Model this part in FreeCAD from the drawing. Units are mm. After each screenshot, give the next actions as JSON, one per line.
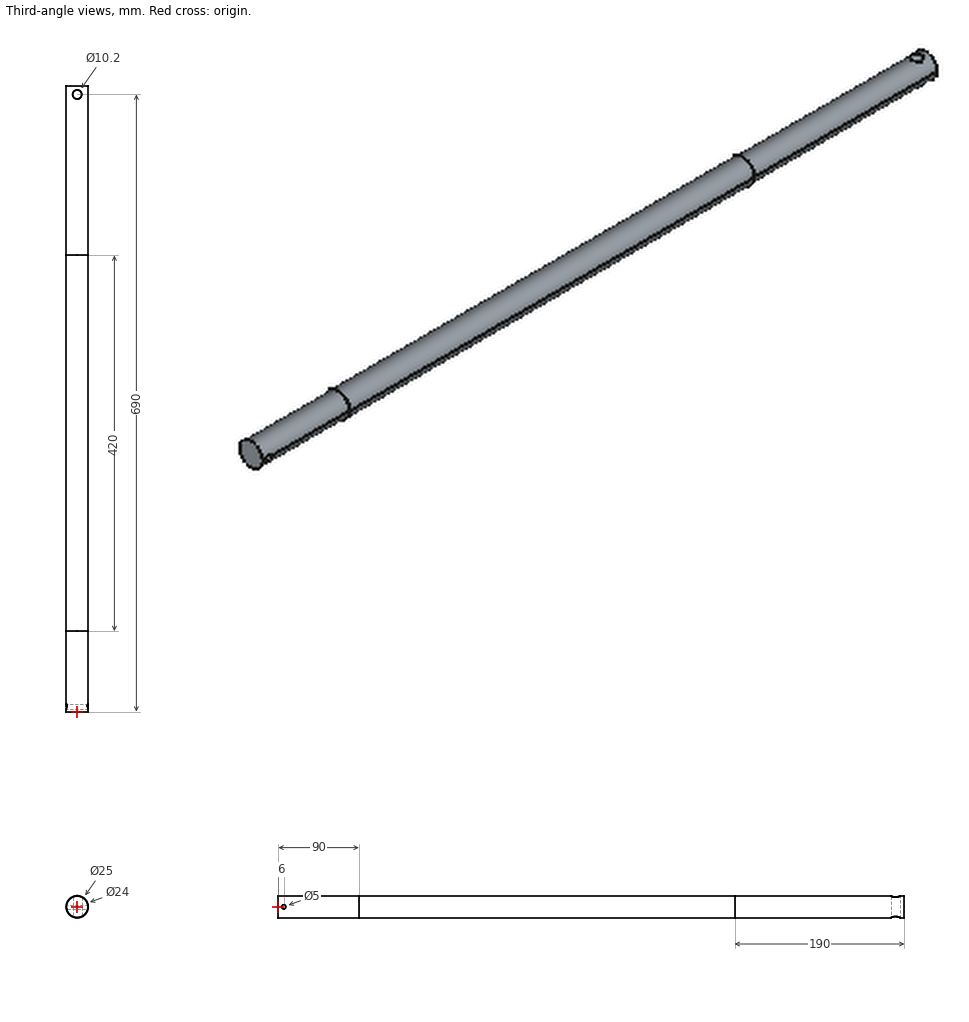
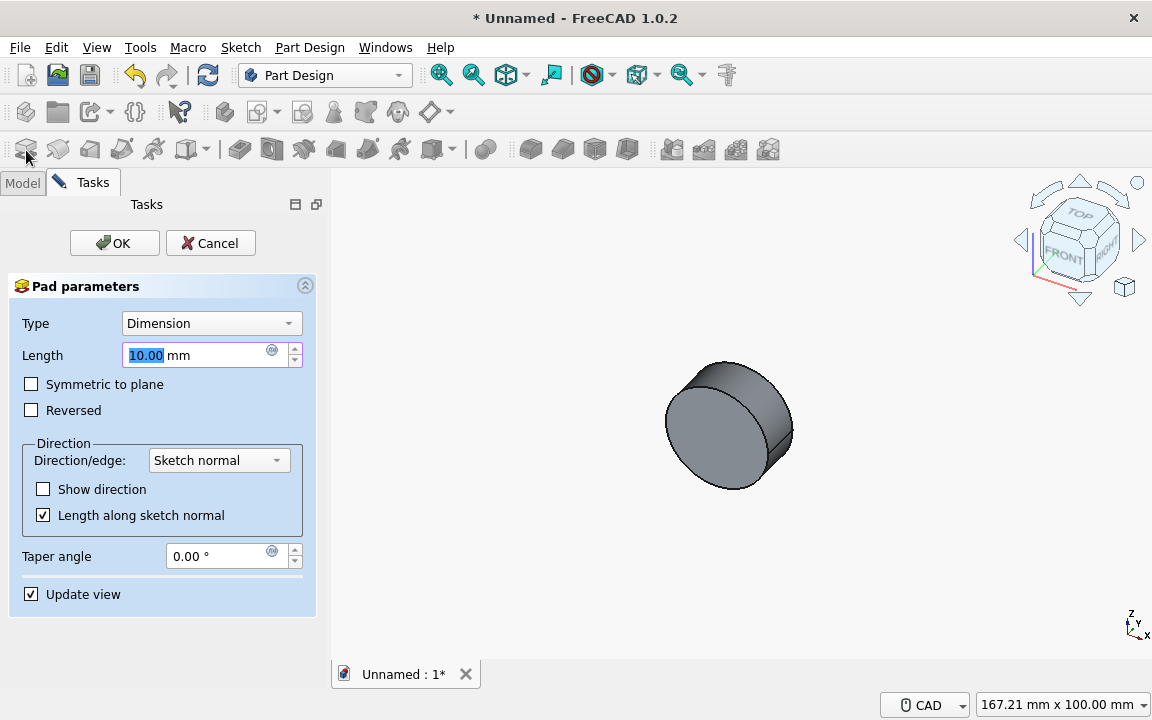
{"action": "type", "text": "90"}
{"action": "key", "text": "Tab"}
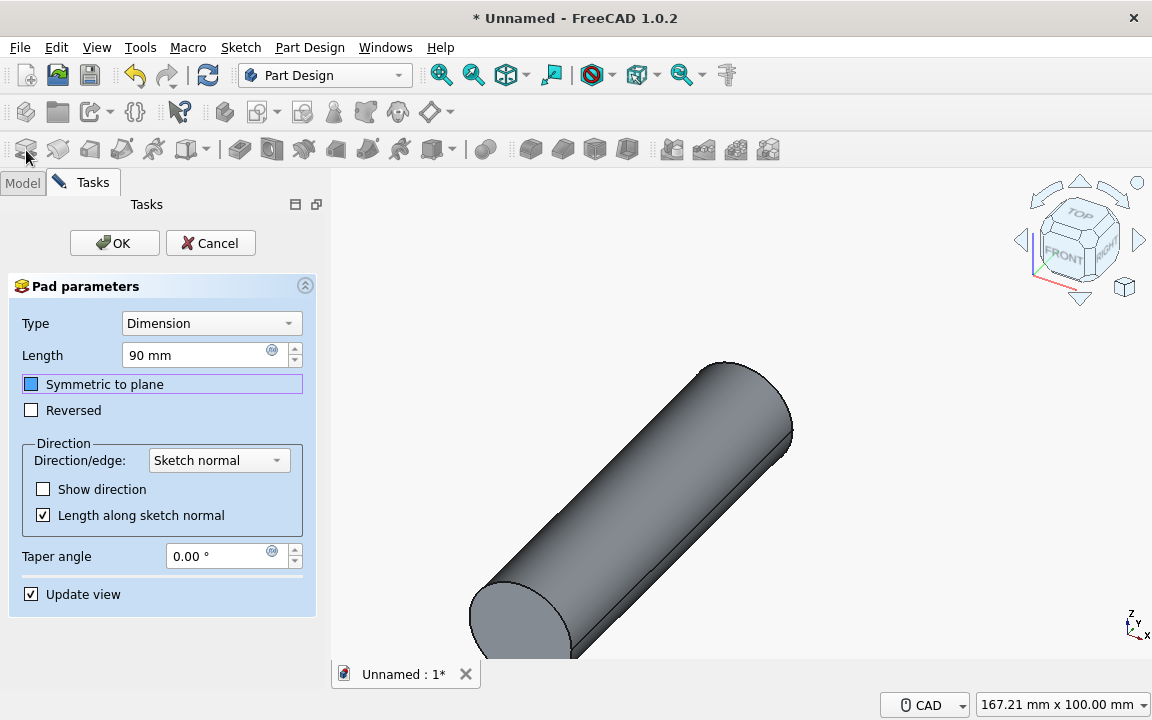
{"action": "left_click", "coordinate": [30, 410]}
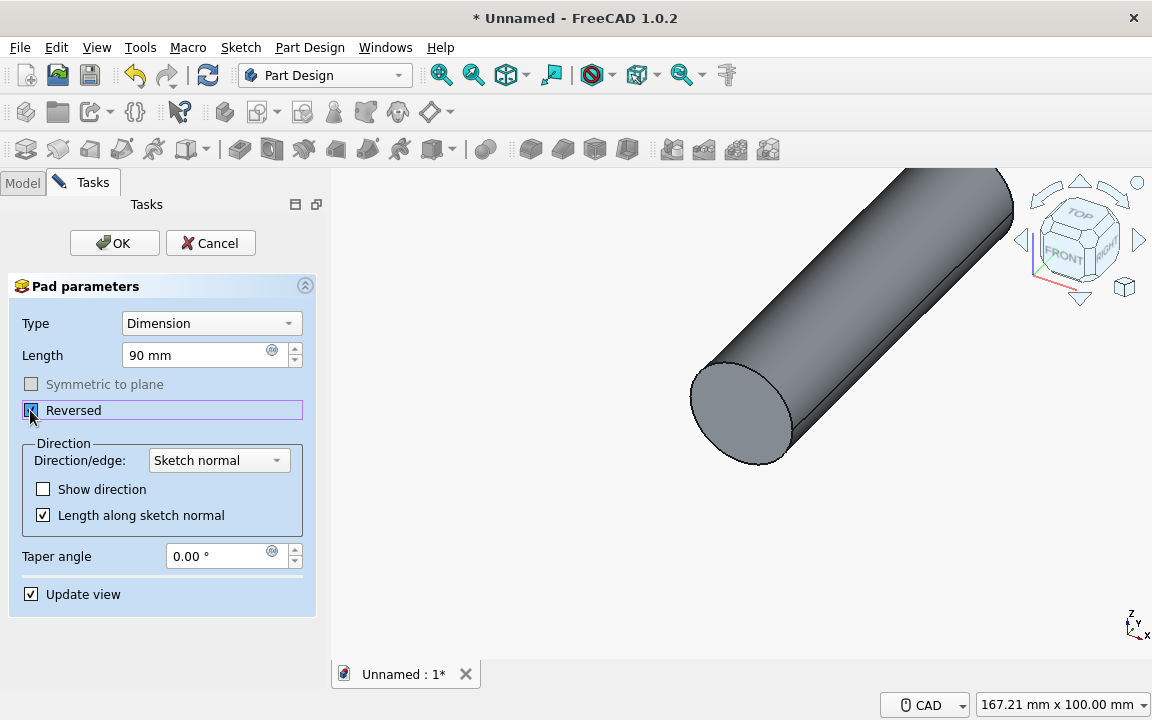
{"action": "left_click", "coordinate": [115, 243]}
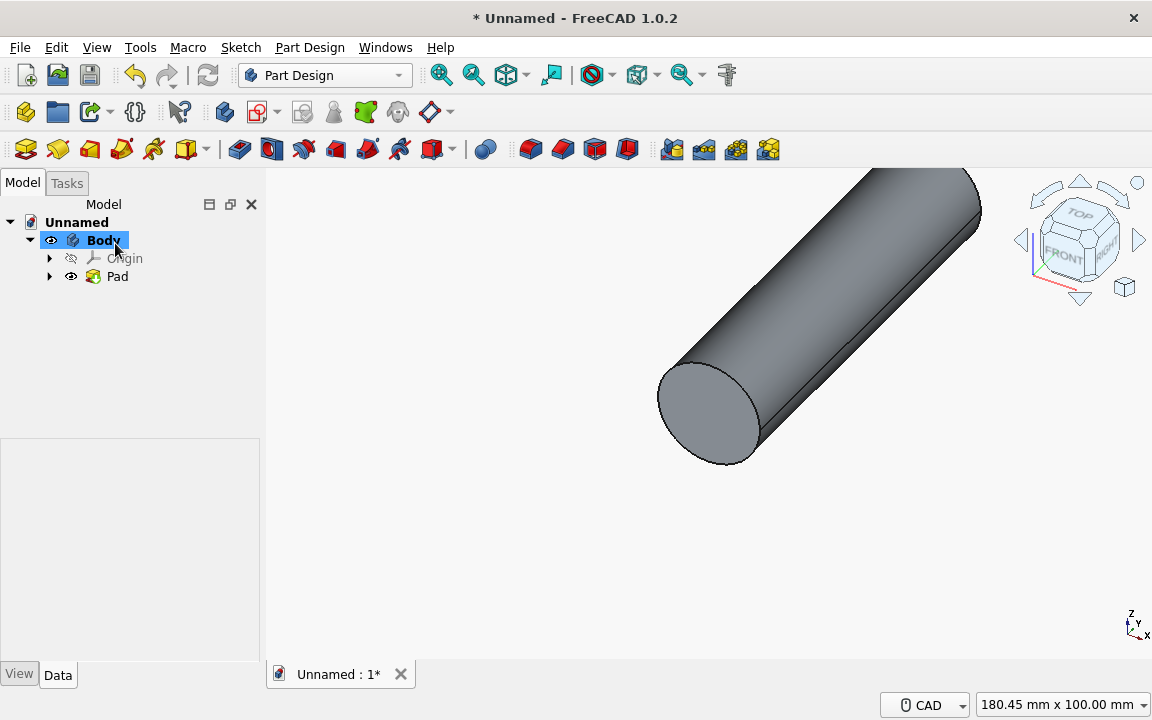
{"action": "left_click", "coordinate": [442, 76]}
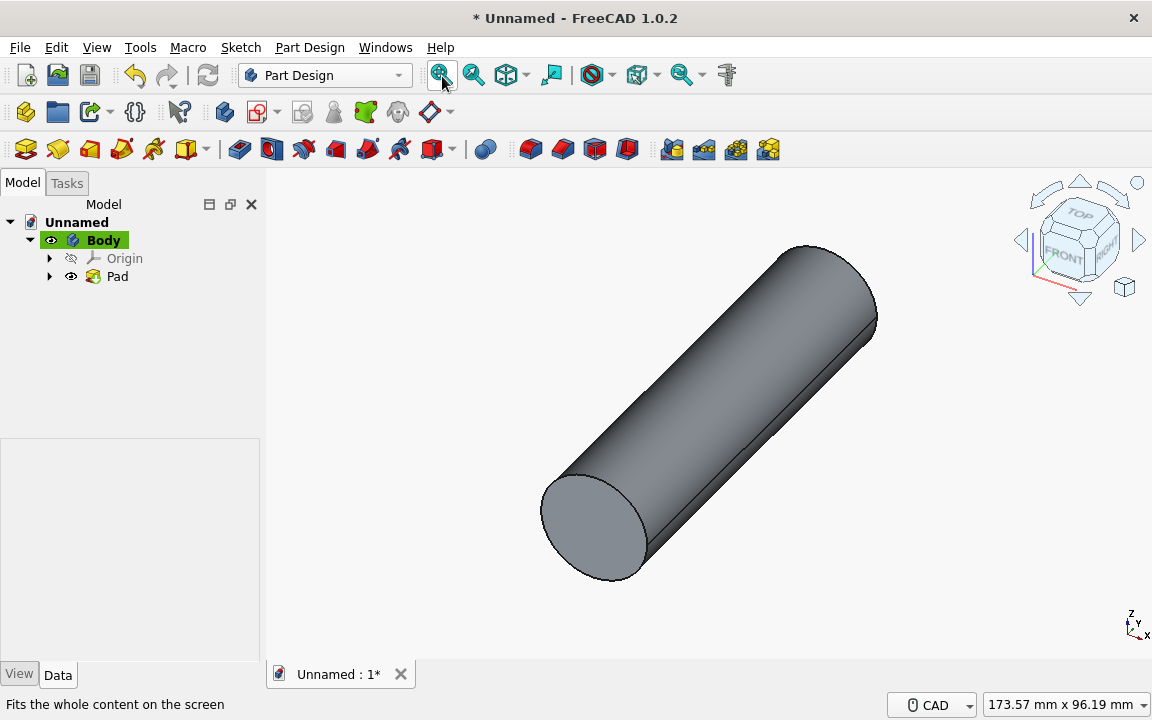
{"action": "key", "text": "4"}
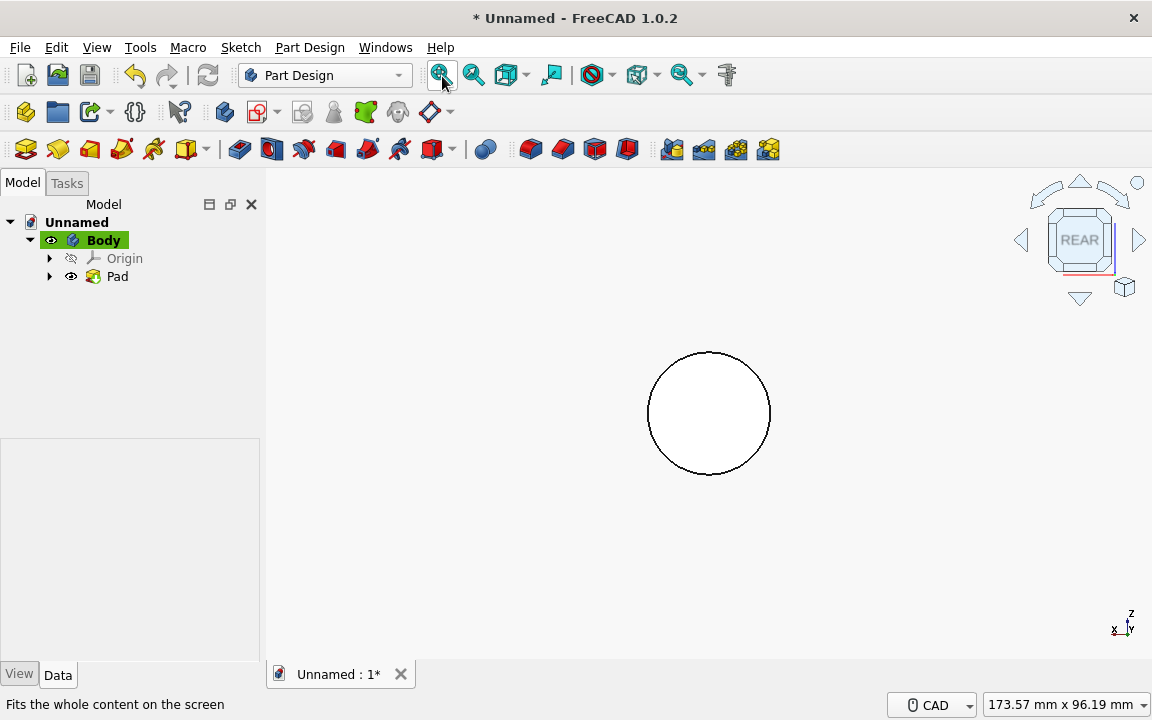
{"action": "left_click", "coordinate": [442, 76]}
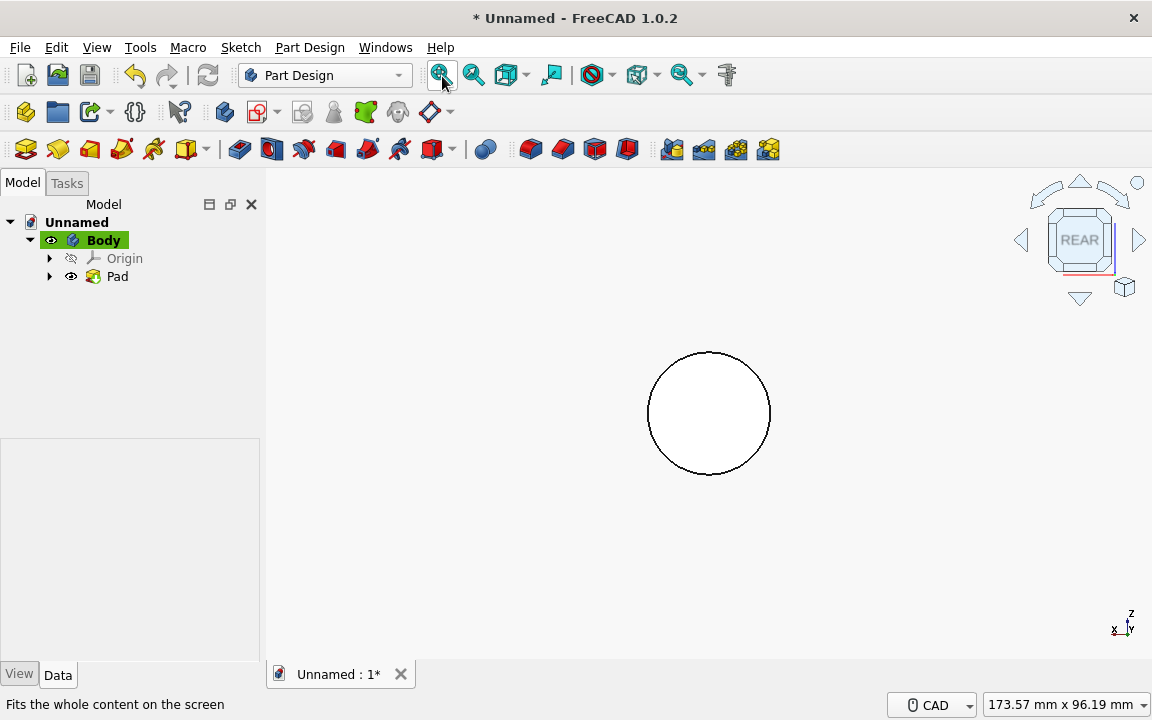
{"action": "left_click", "coordinate": [709, 413]}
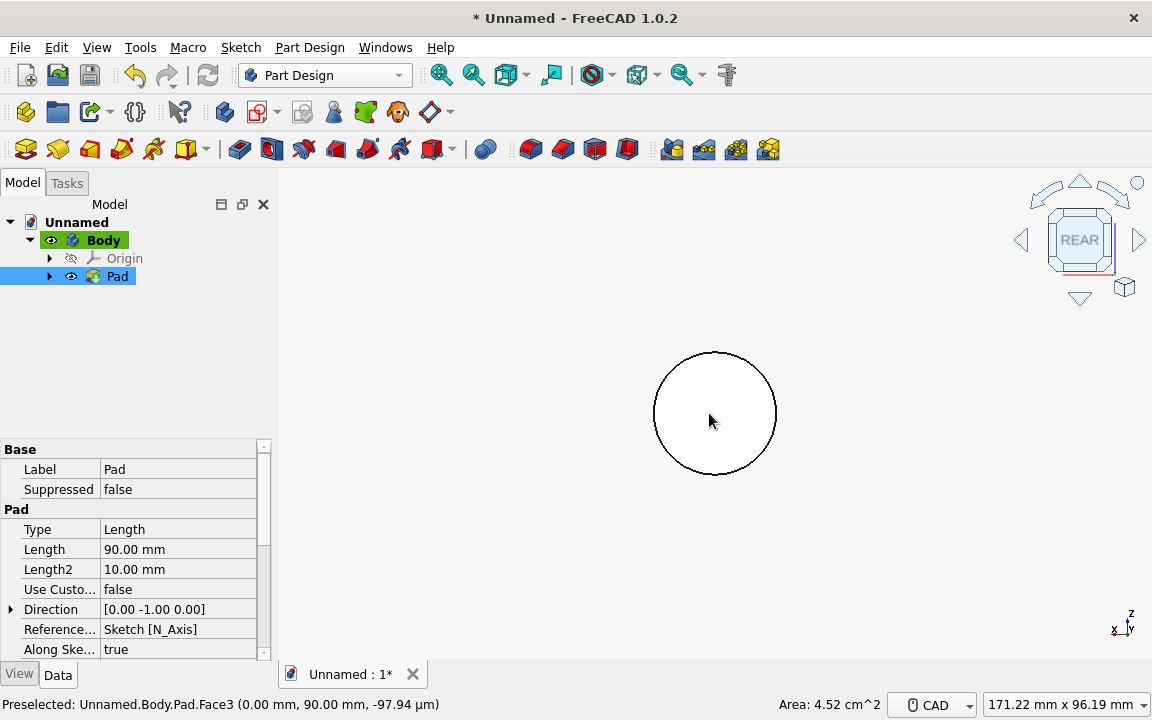
{"action": "left_click", "coordinate": [258, 112]}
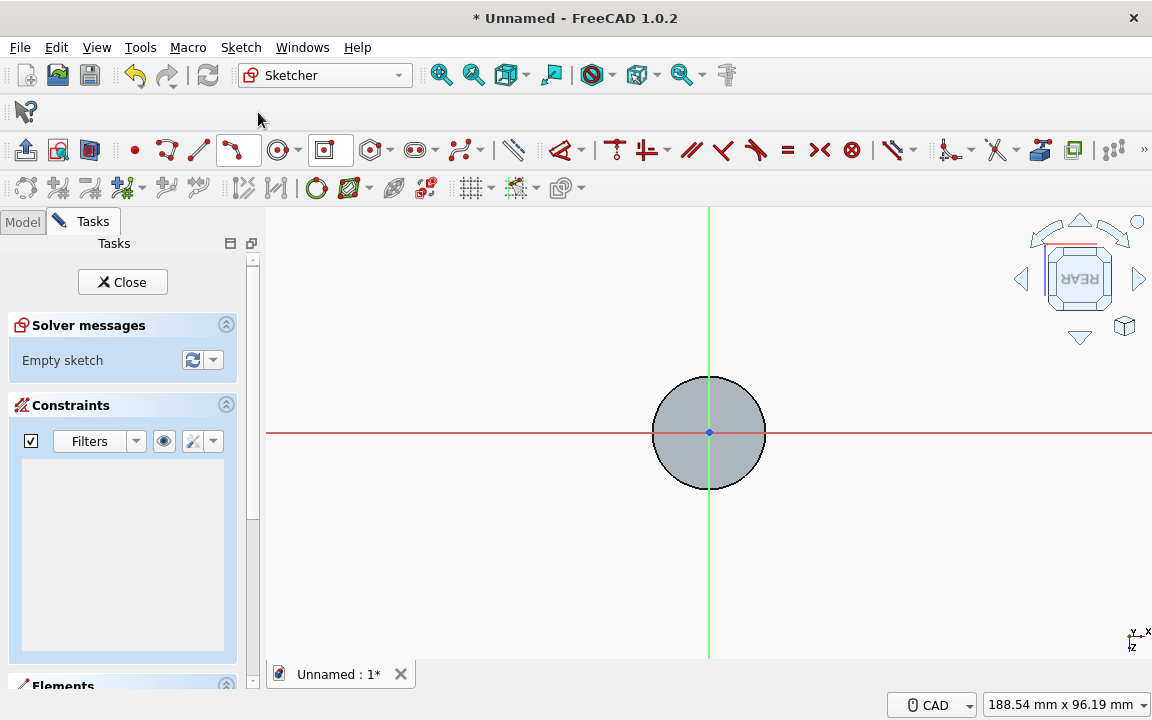
{"action": "scroll", "coordinate": [765, 433], "scroll_direction": "up", "scroll_amount": 4}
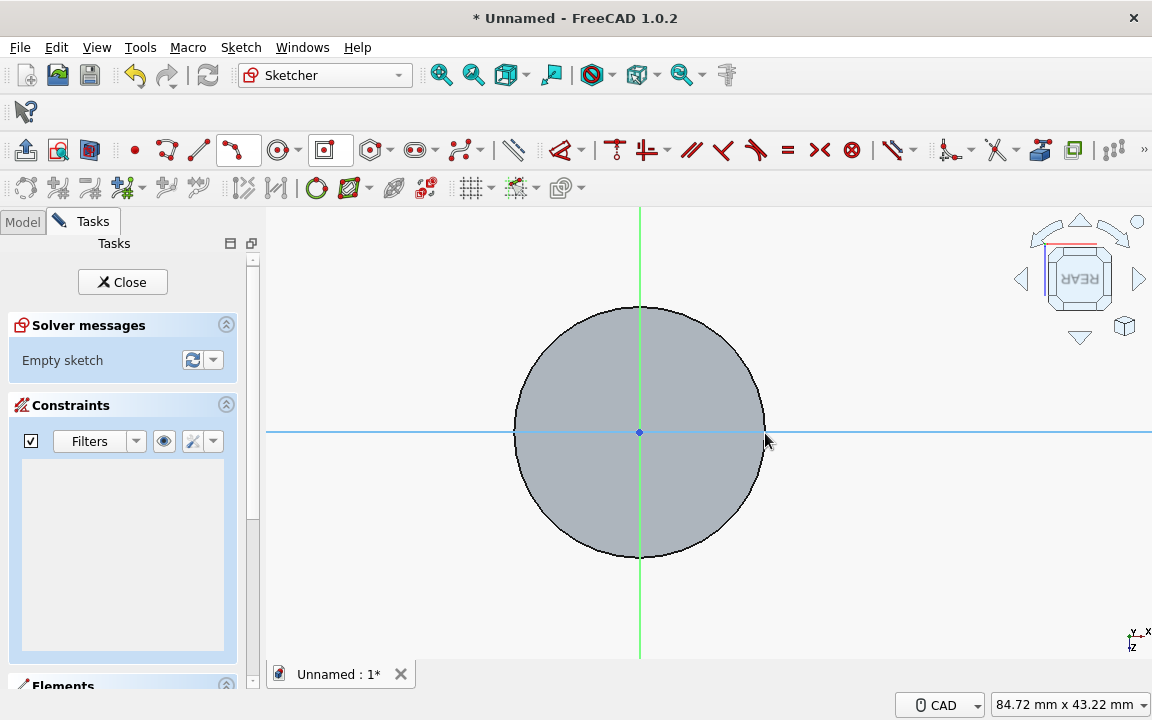
{"action": "left_click", "coordinate": [278, 150]}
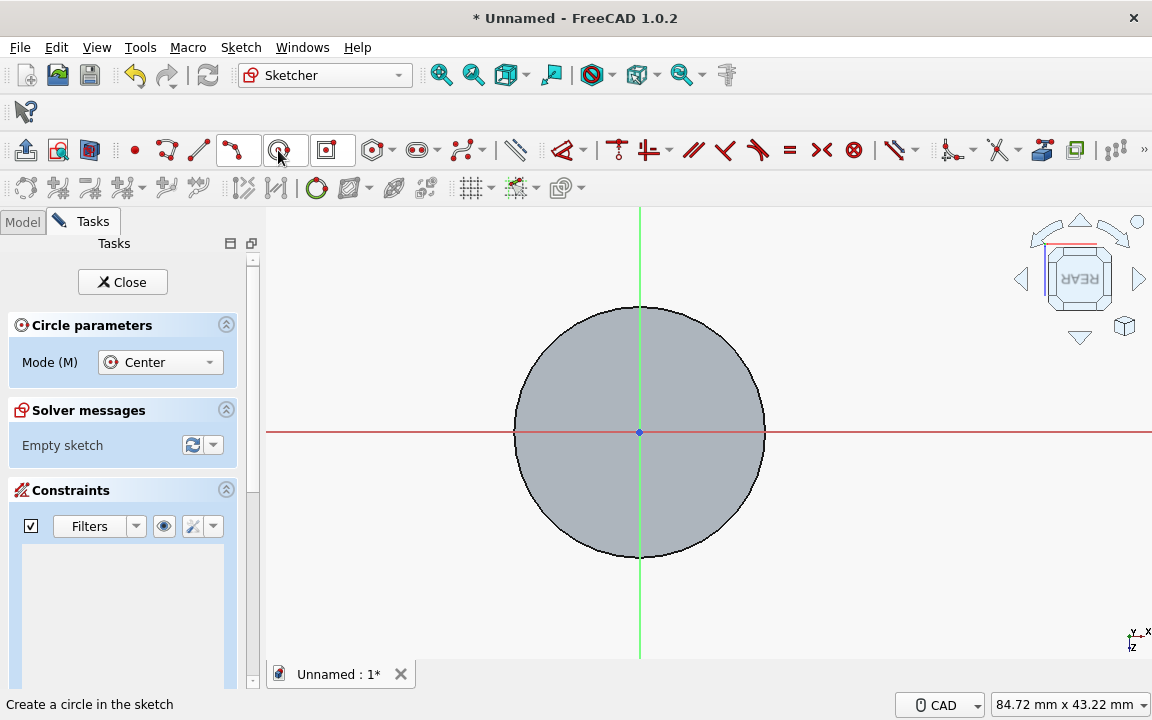
{"action": "left_click", "coordinate": [640, 432]}
{"action": "left_click", "coordinate": [732, 340]}
{"action": "key", "text": "Escape"}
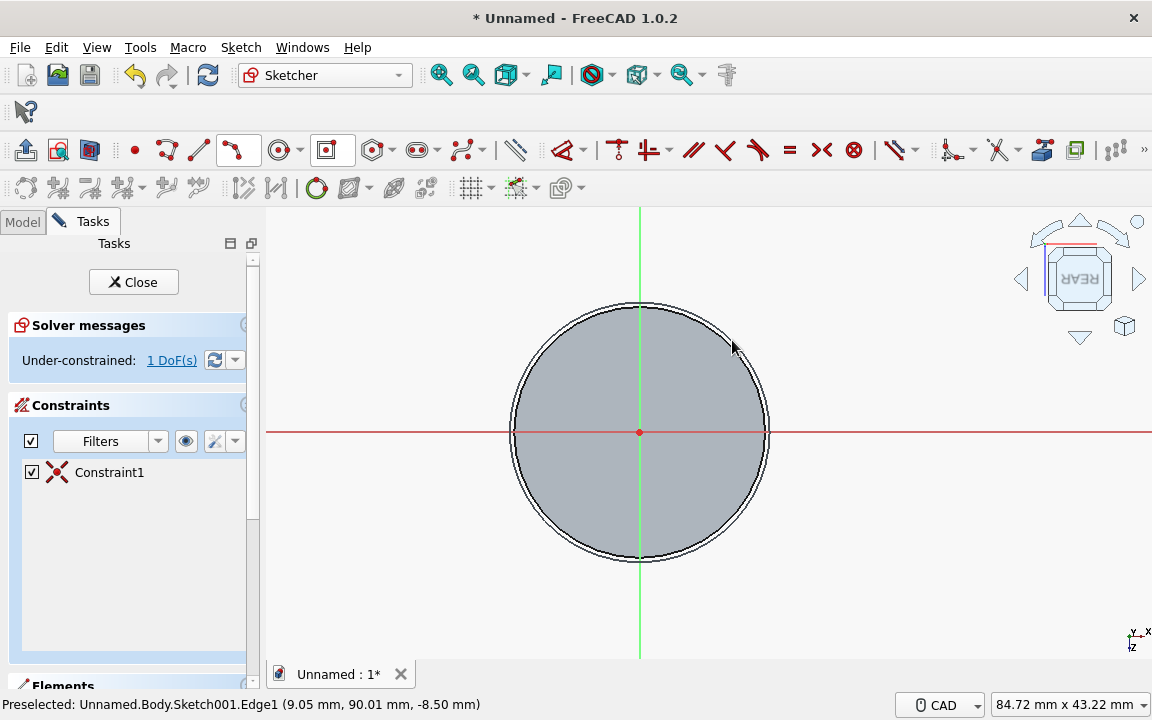
{"action": "left_click", "coordinate": [731, 340]}